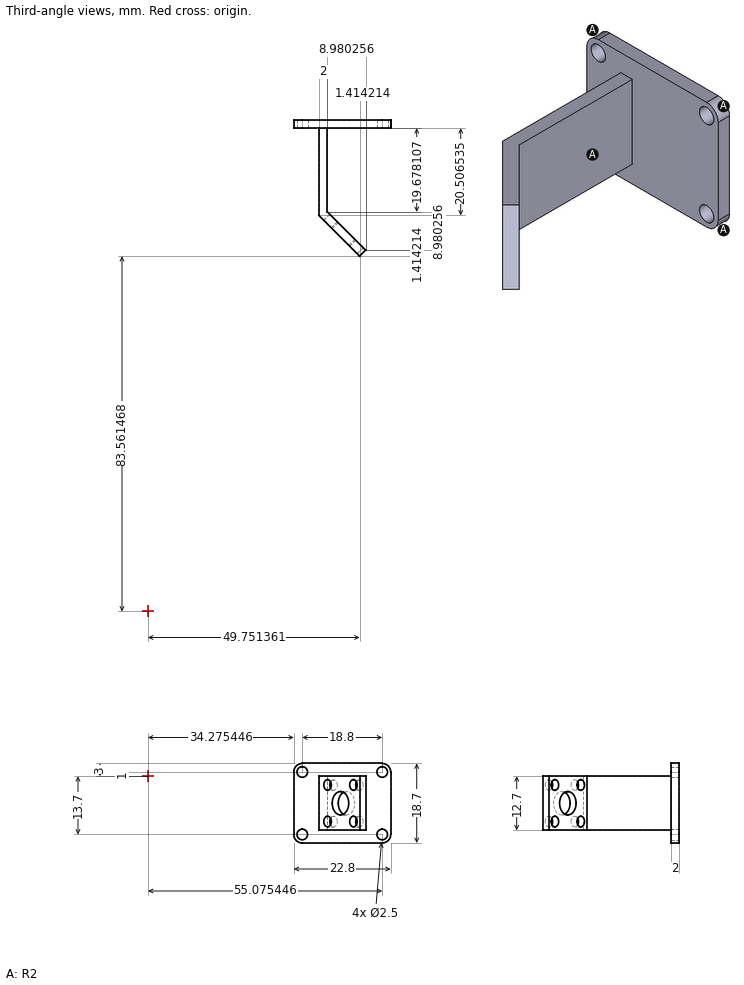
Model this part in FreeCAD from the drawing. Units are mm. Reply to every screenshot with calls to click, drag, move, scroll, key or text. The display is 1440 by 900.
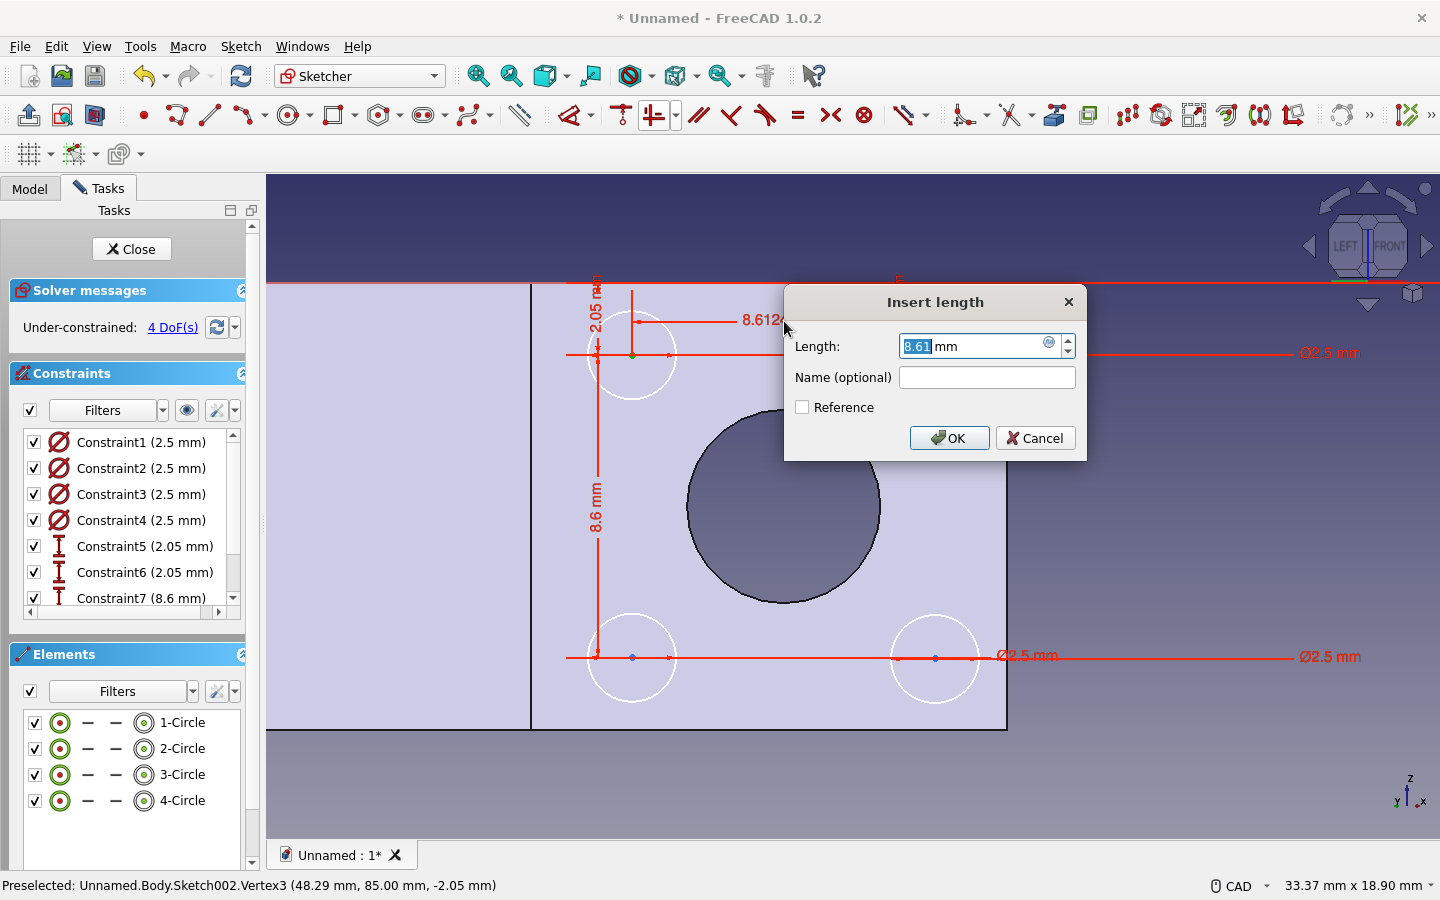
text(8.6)
key(Return)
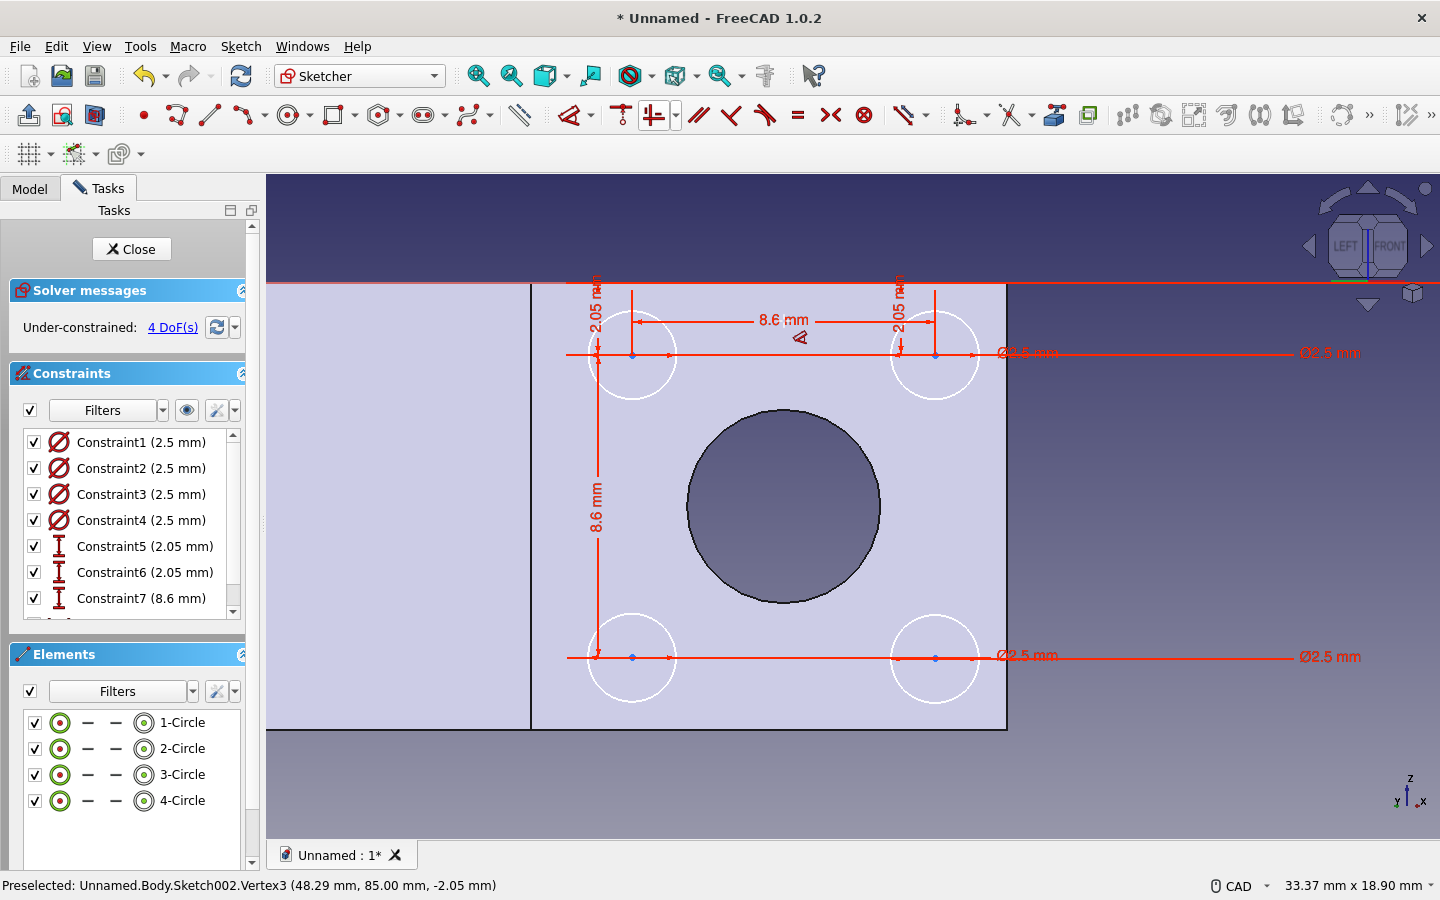
click(632, 658)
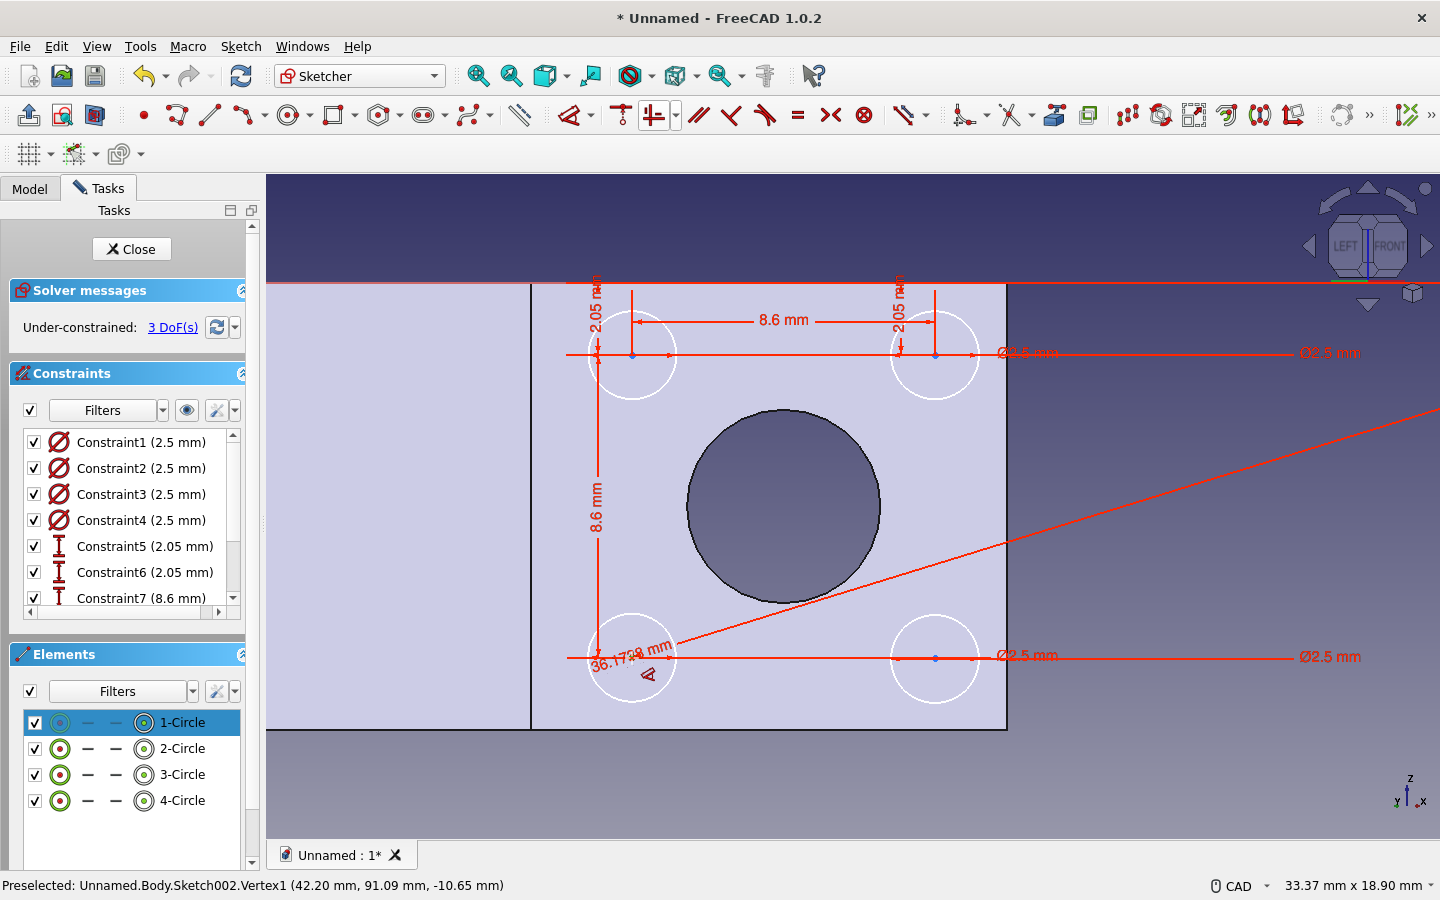
click(935, 355)
click(784, 692)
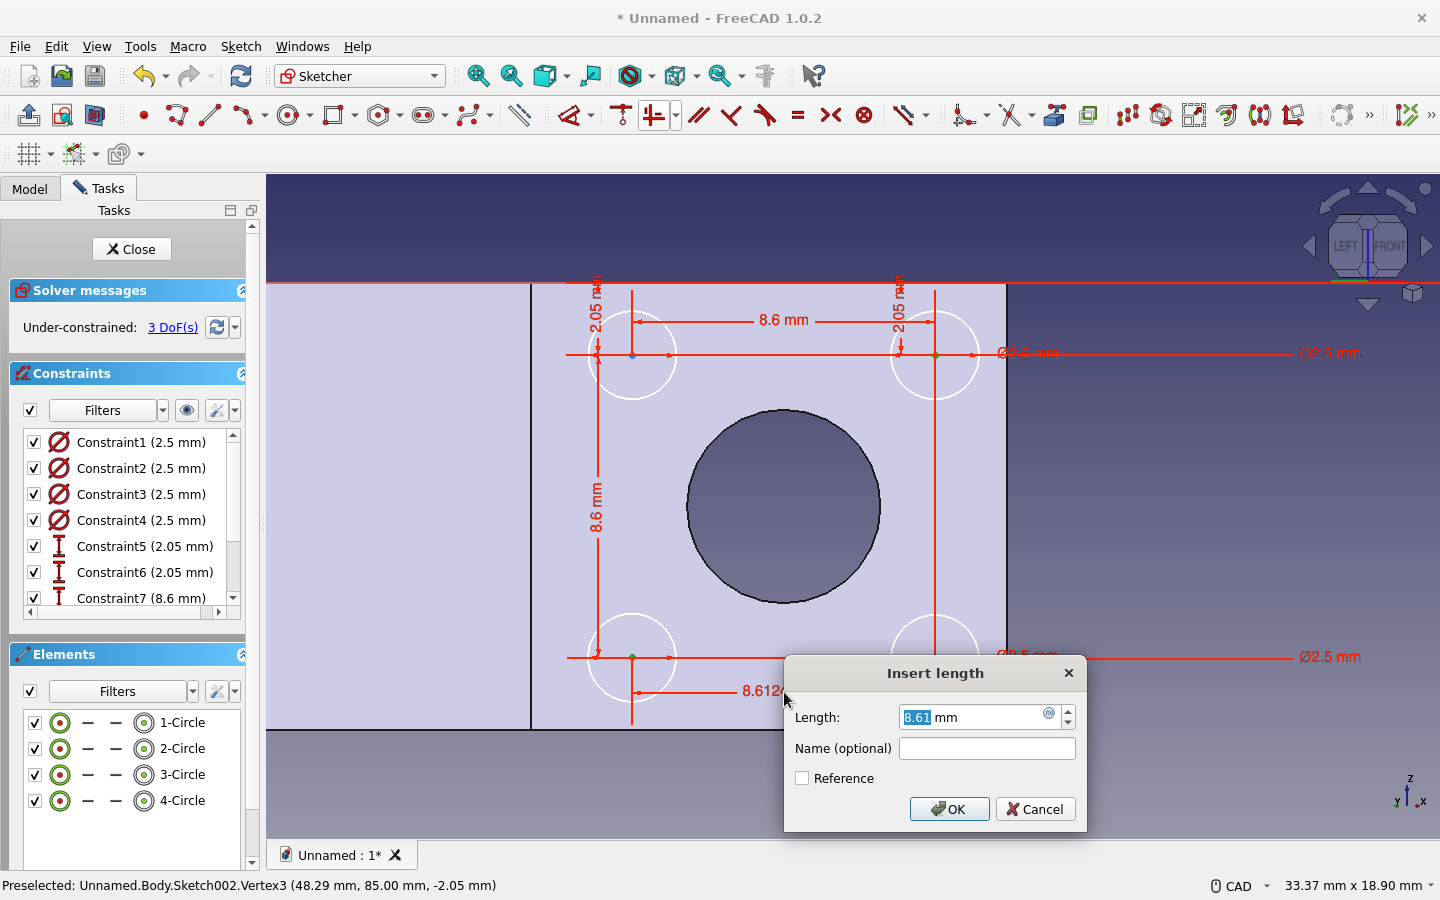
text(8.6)
key(Return)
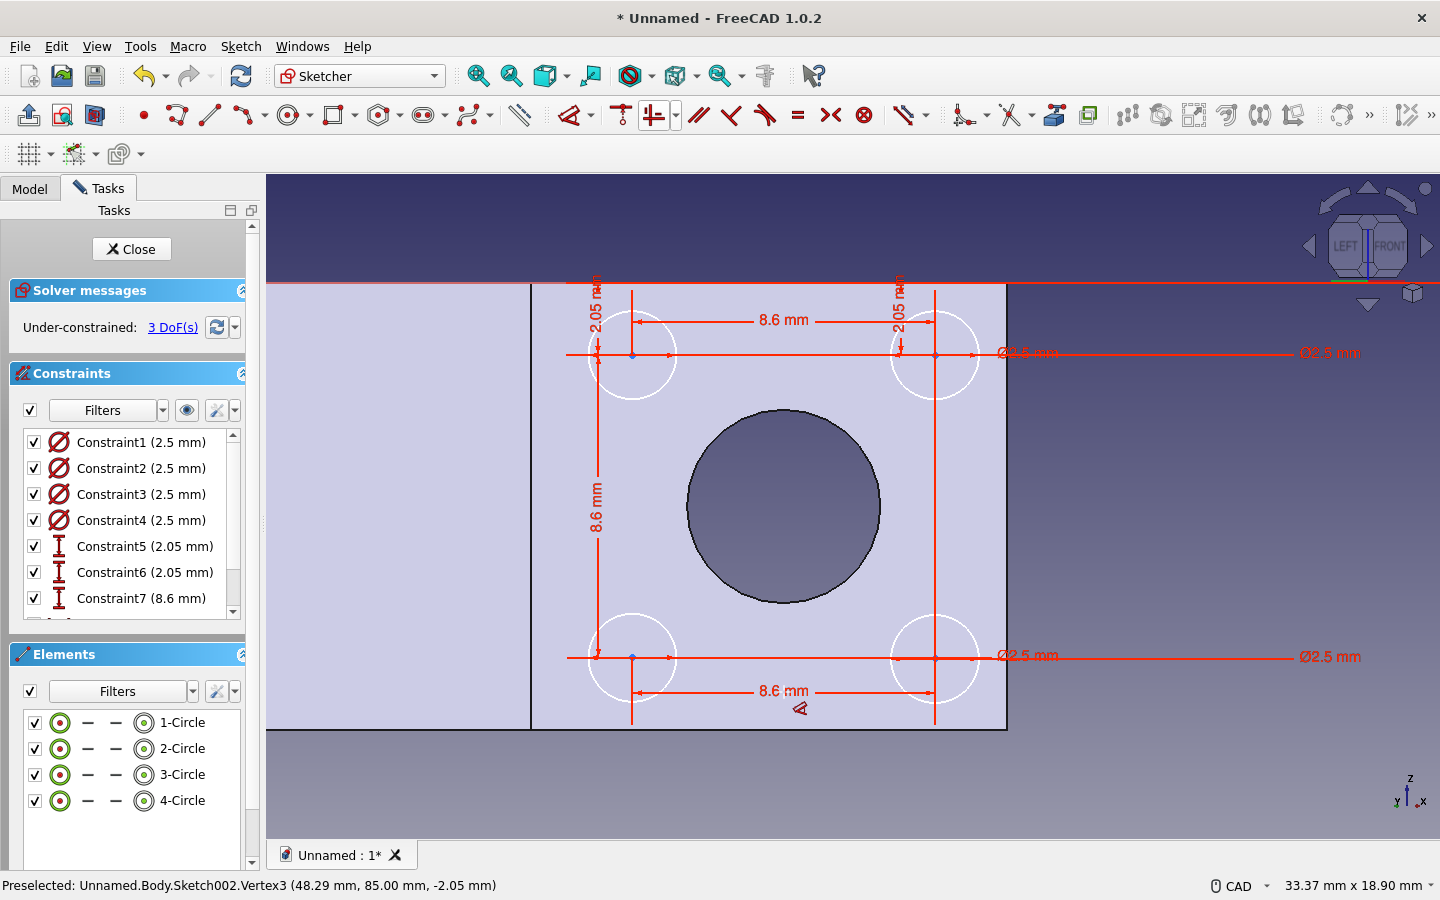
click(632, 658)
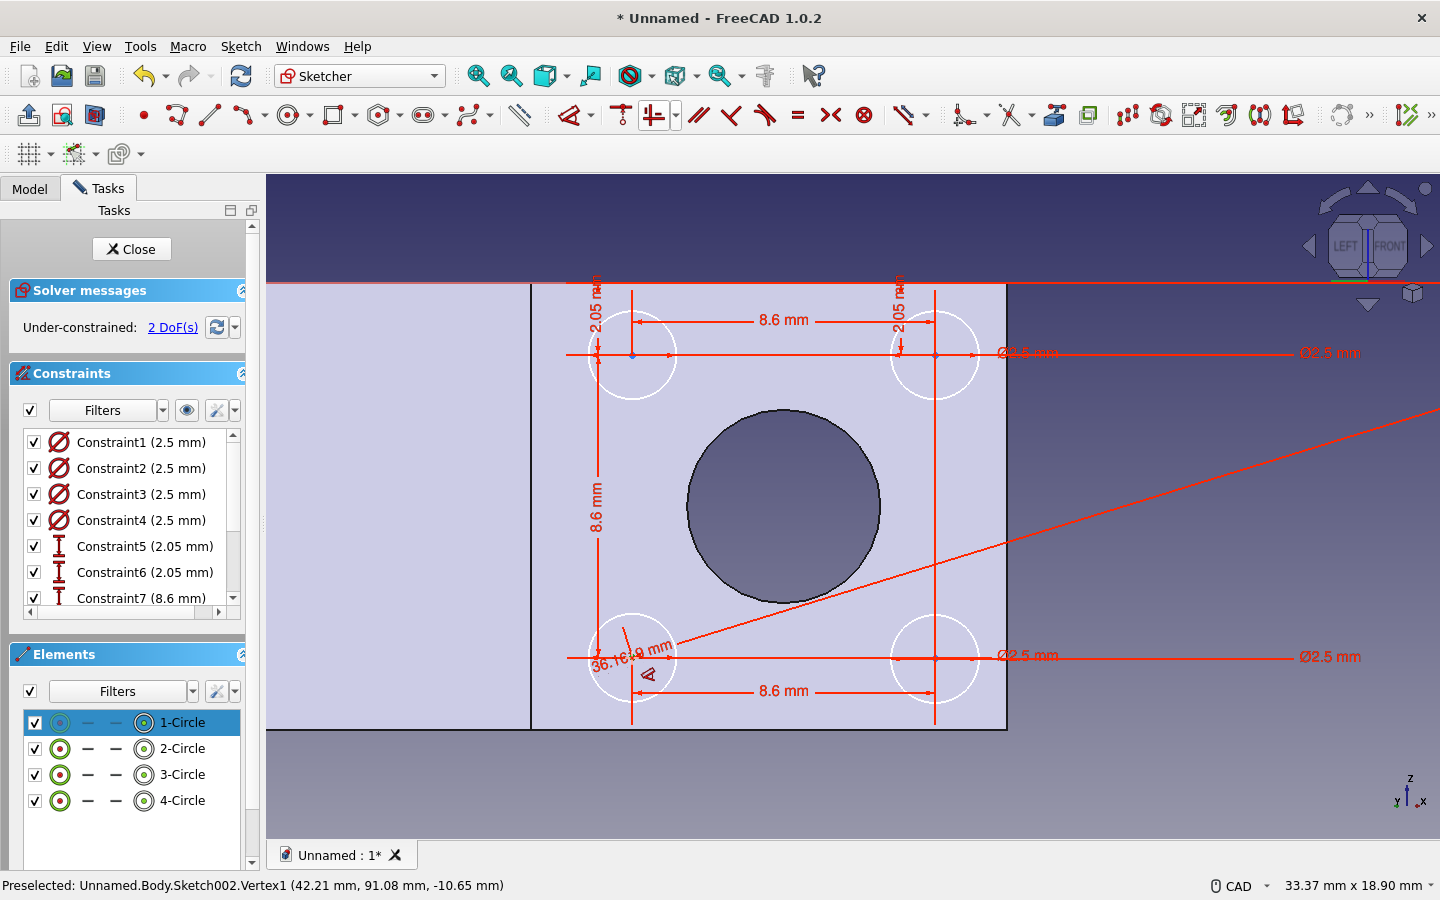
click(935, 659)
click(678, 693)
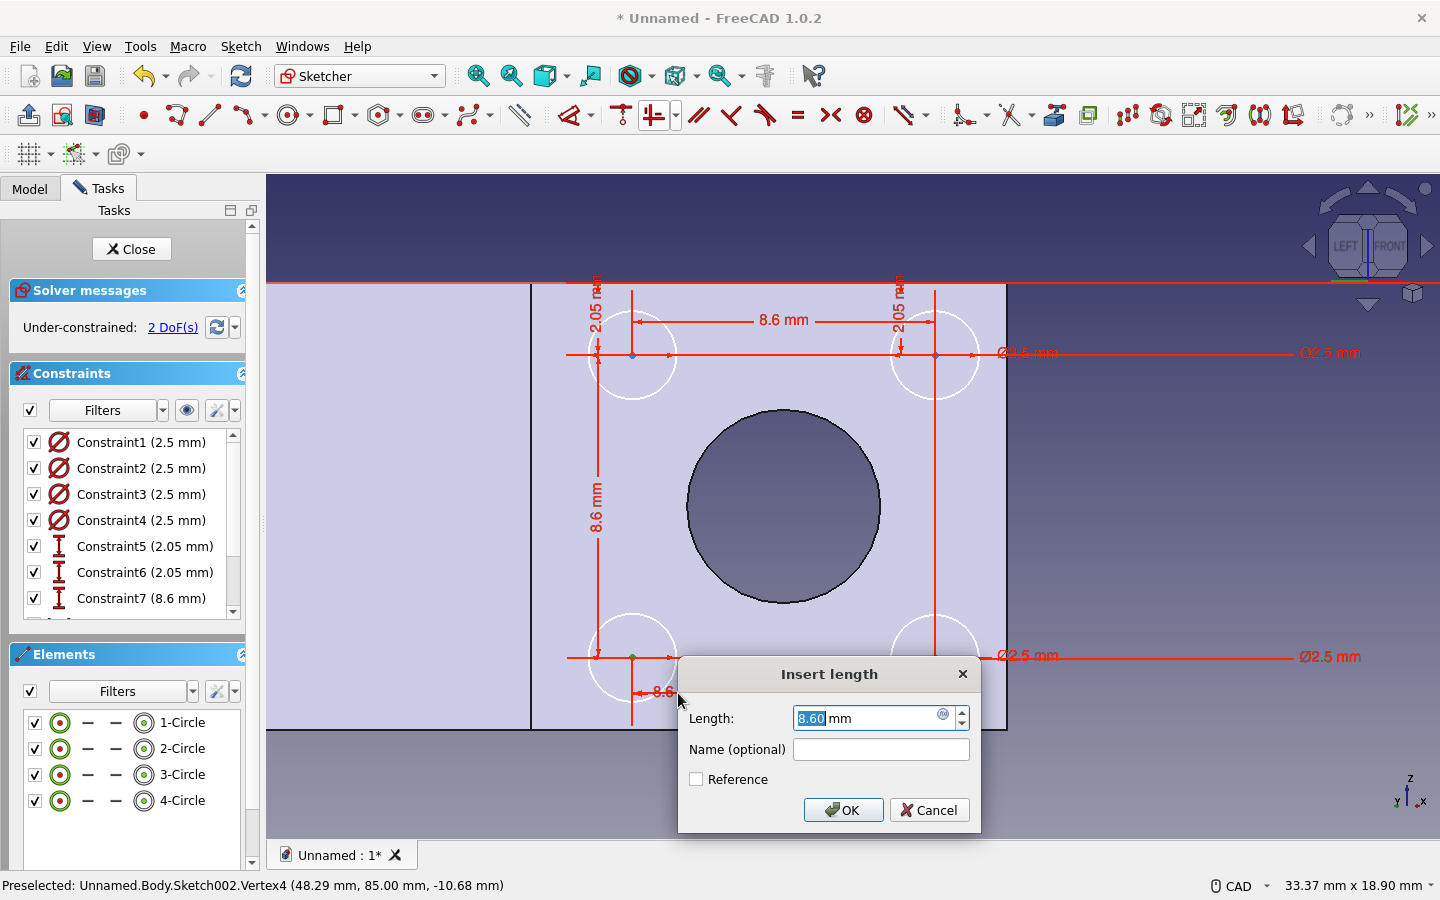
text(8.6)
key(Return)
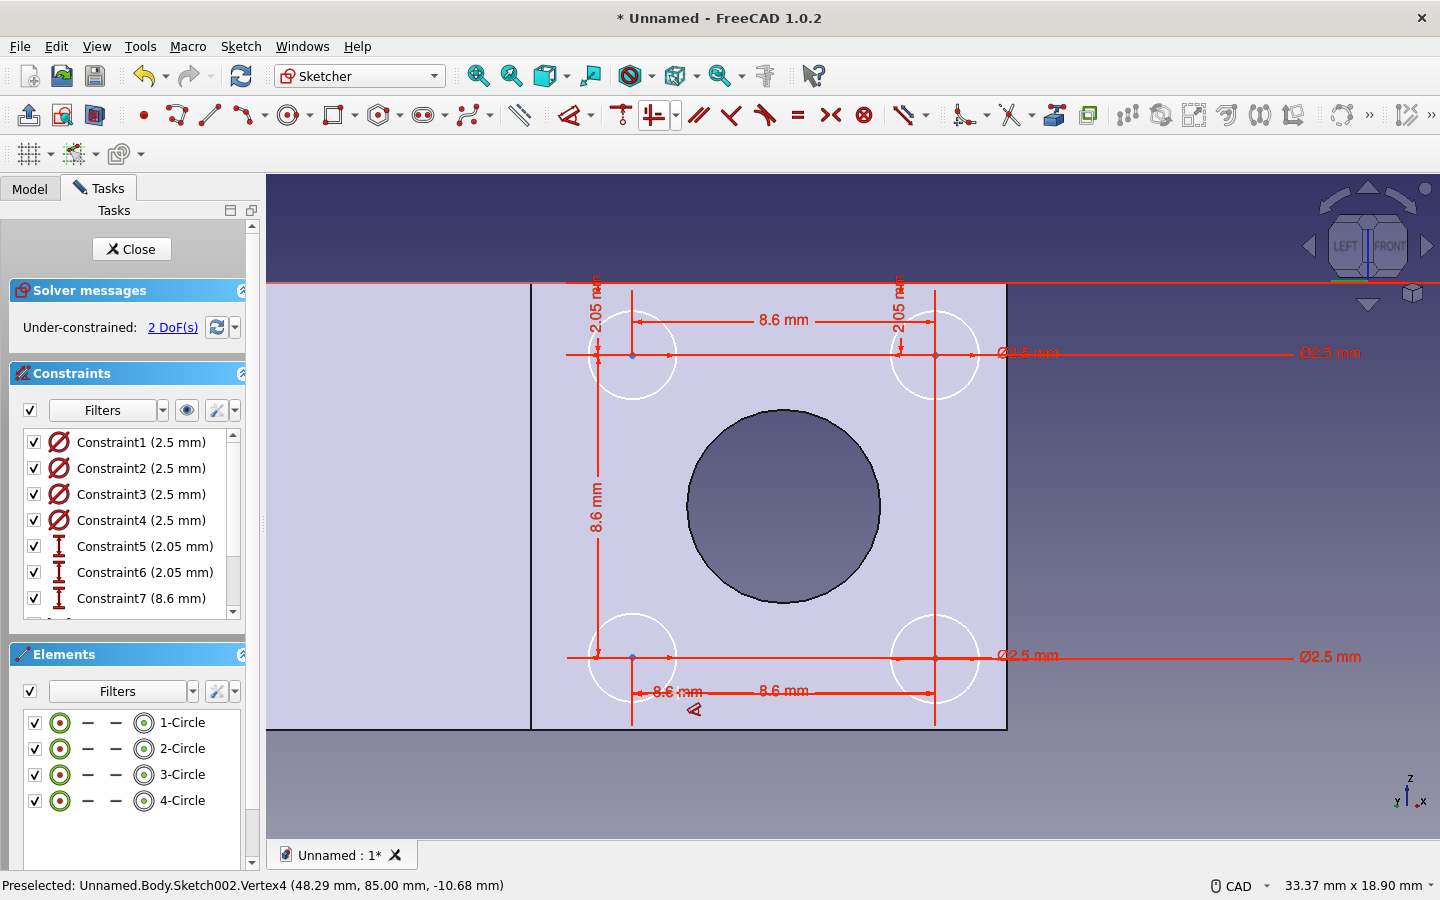
click(935, 355)